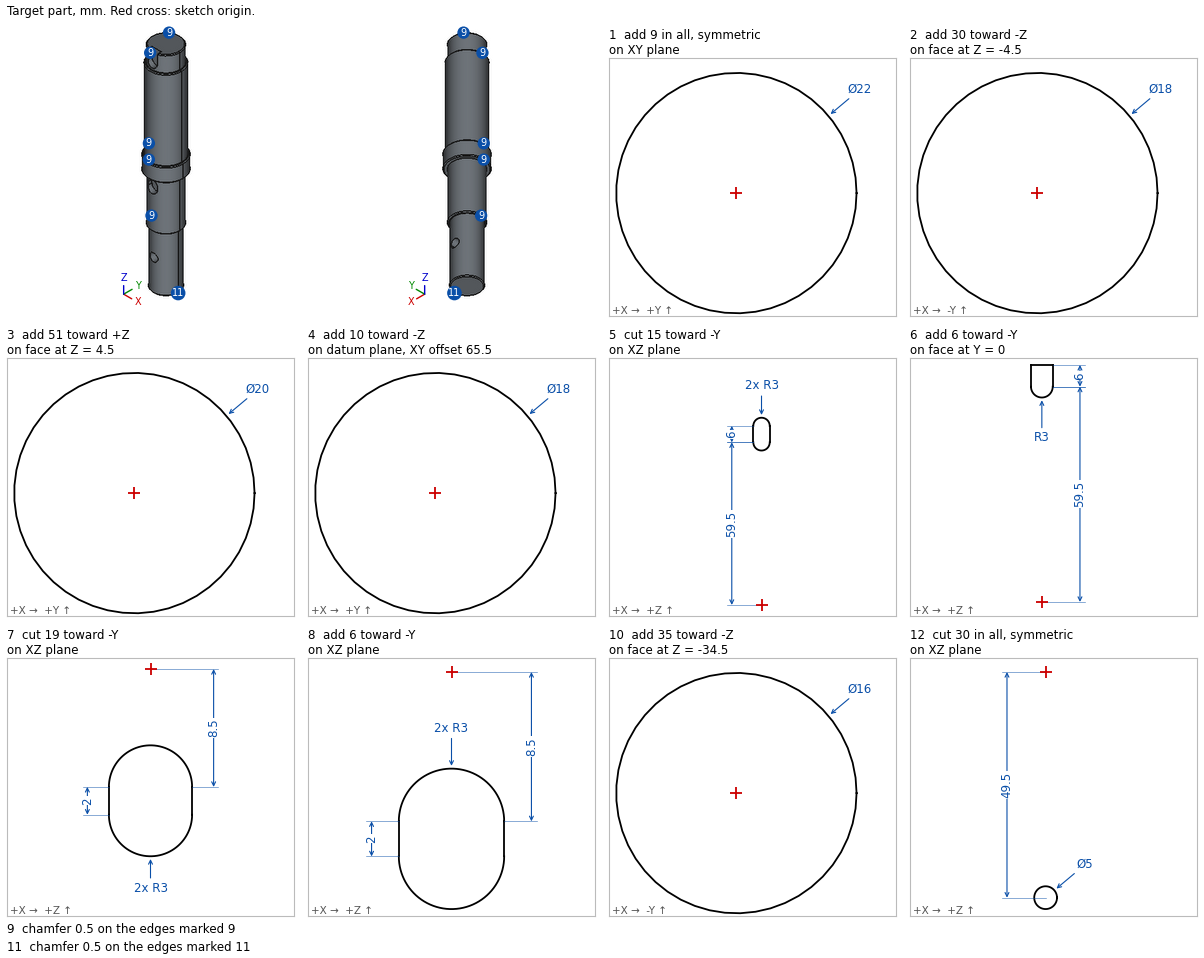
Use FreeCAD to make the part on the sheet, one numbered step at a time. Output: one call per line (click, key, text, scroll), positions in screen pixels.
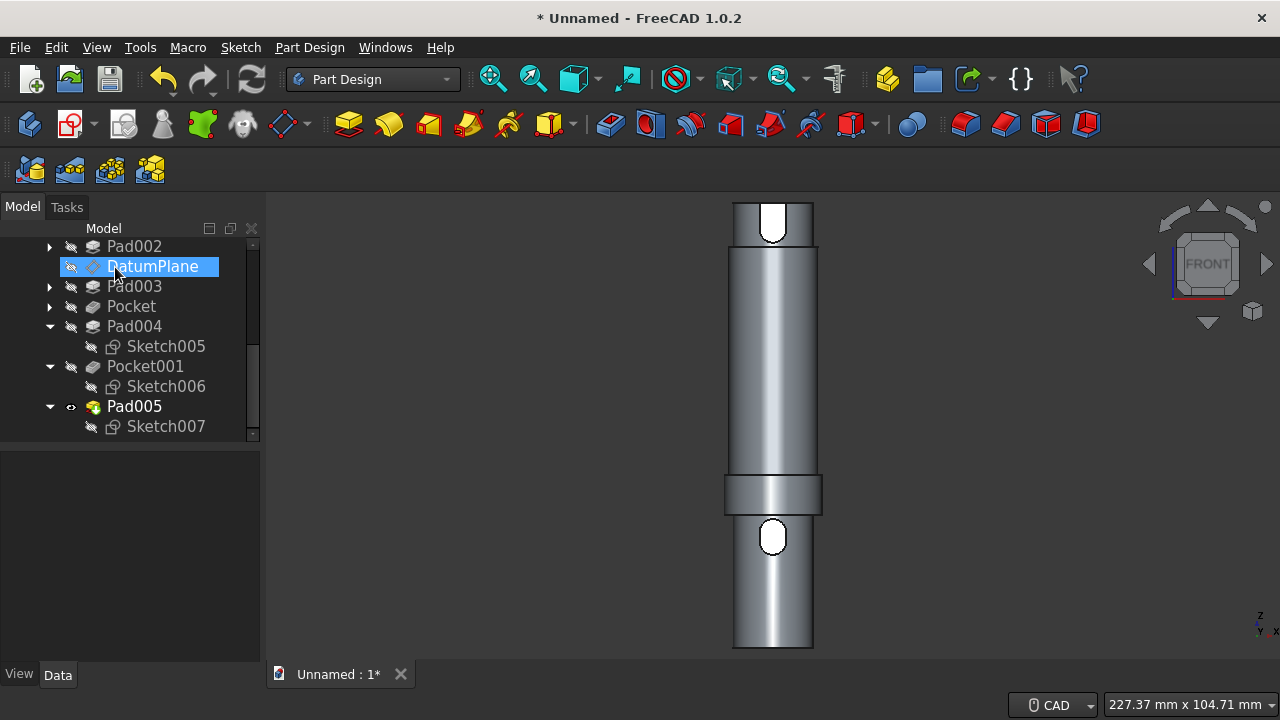
click(737, 246)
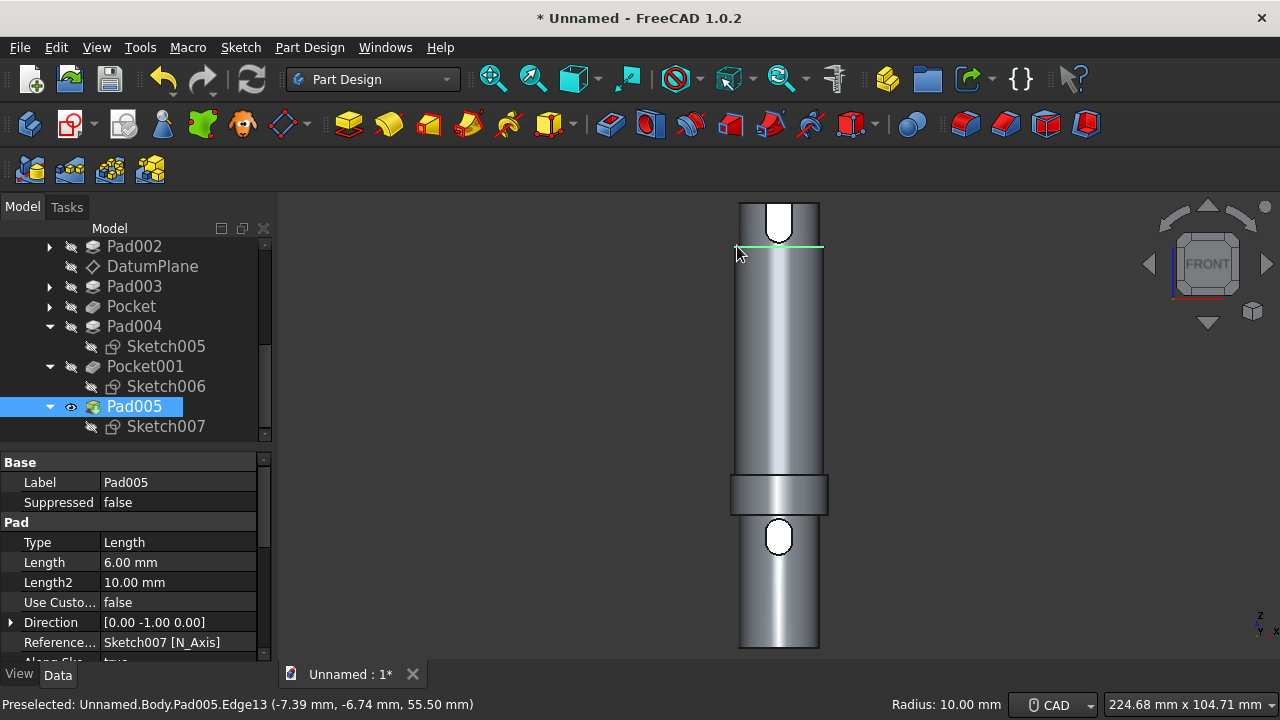
click(739, 514, ctrl)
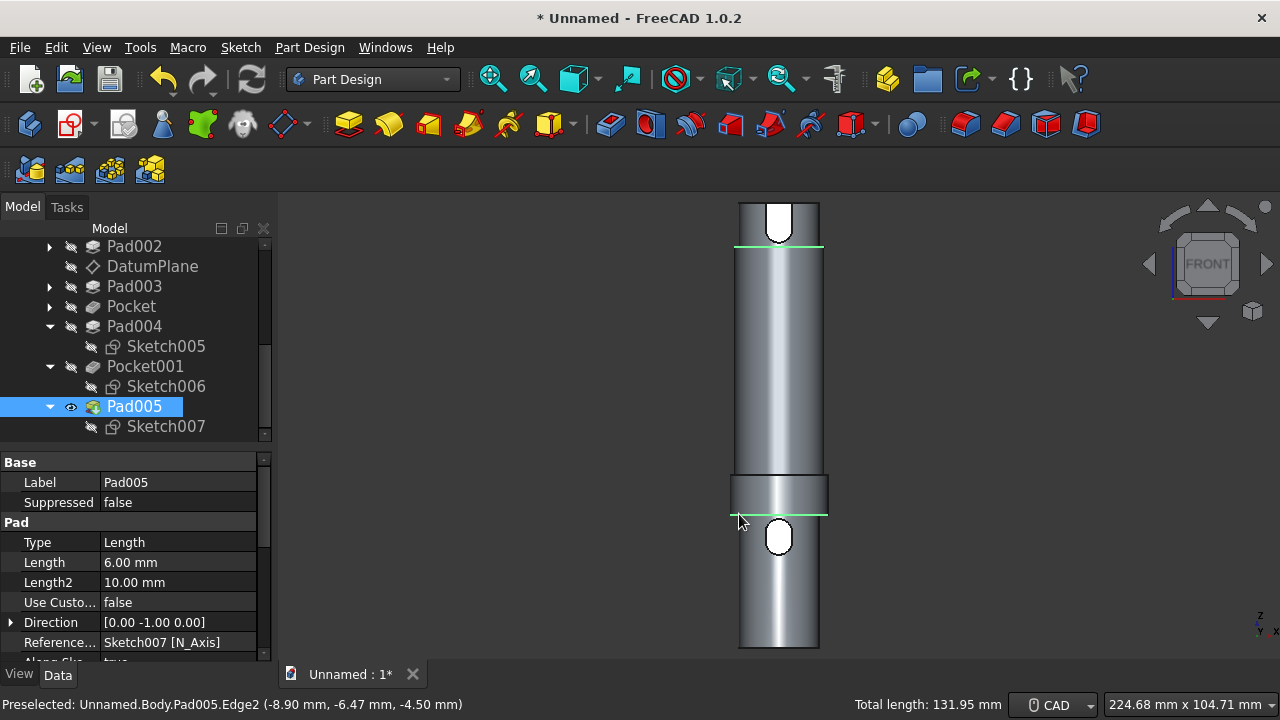
click(739, 474, ctrl)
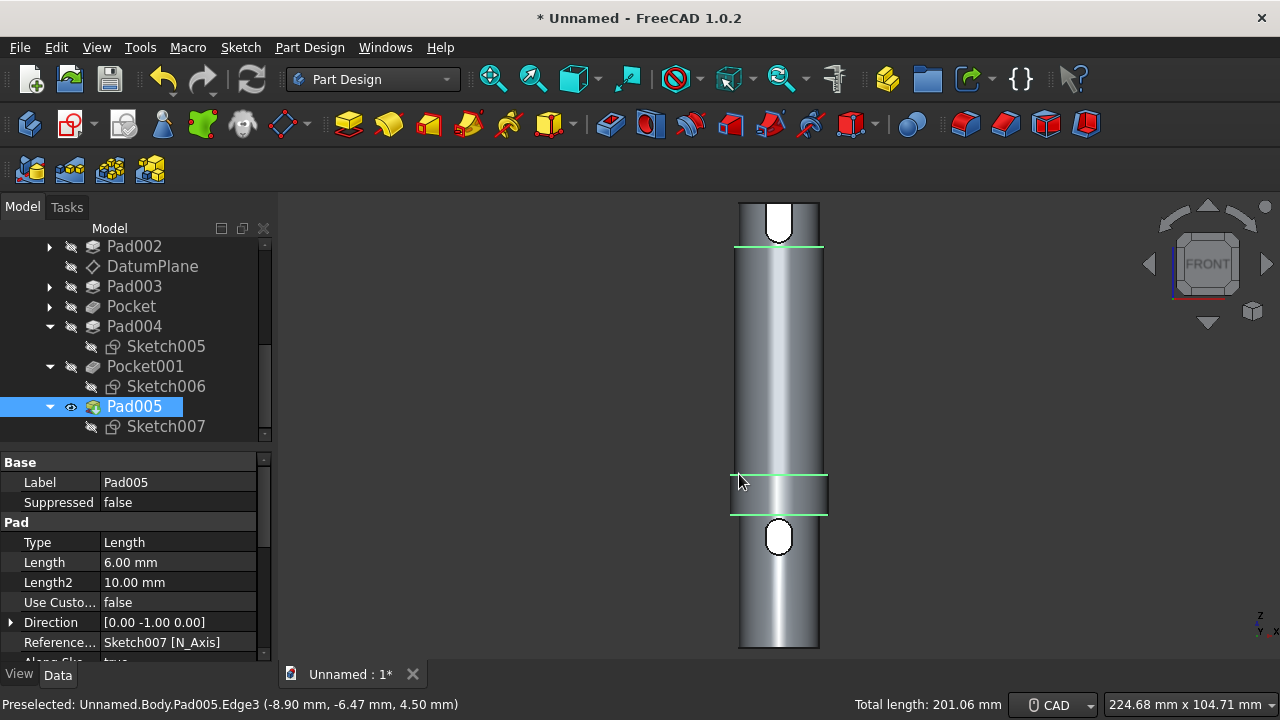
key(0)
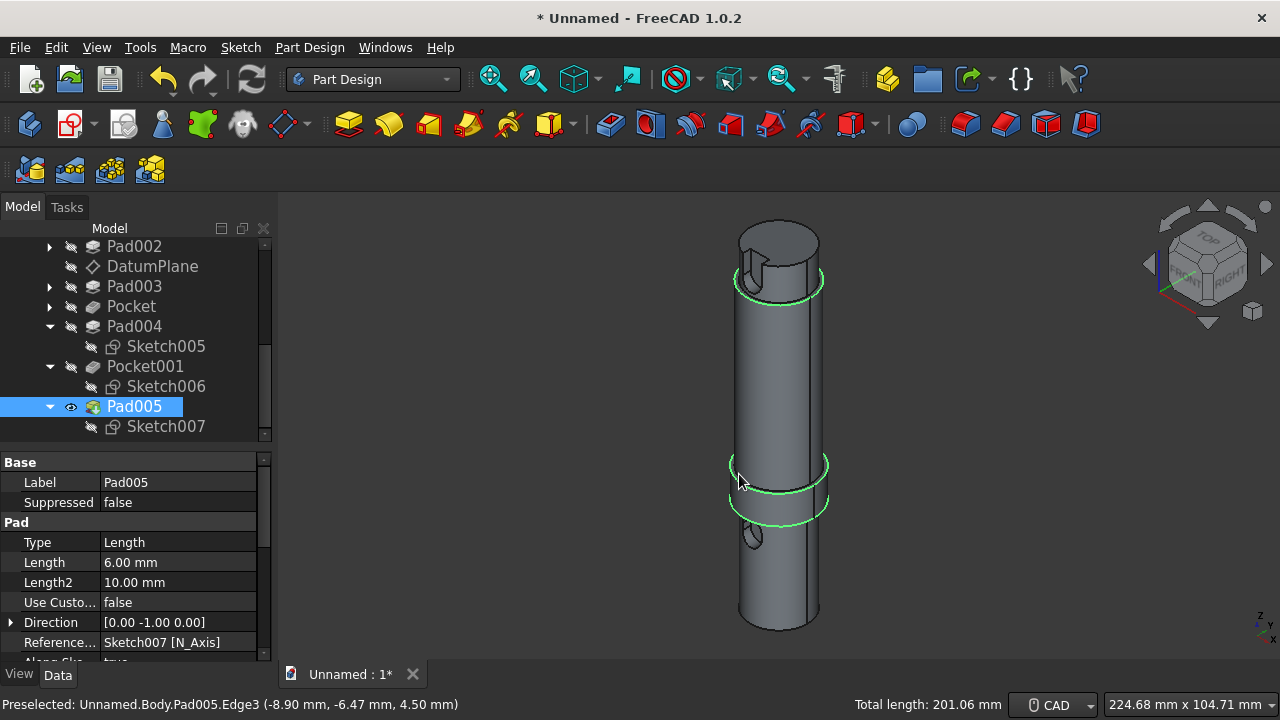
click(814, 231, ctrl)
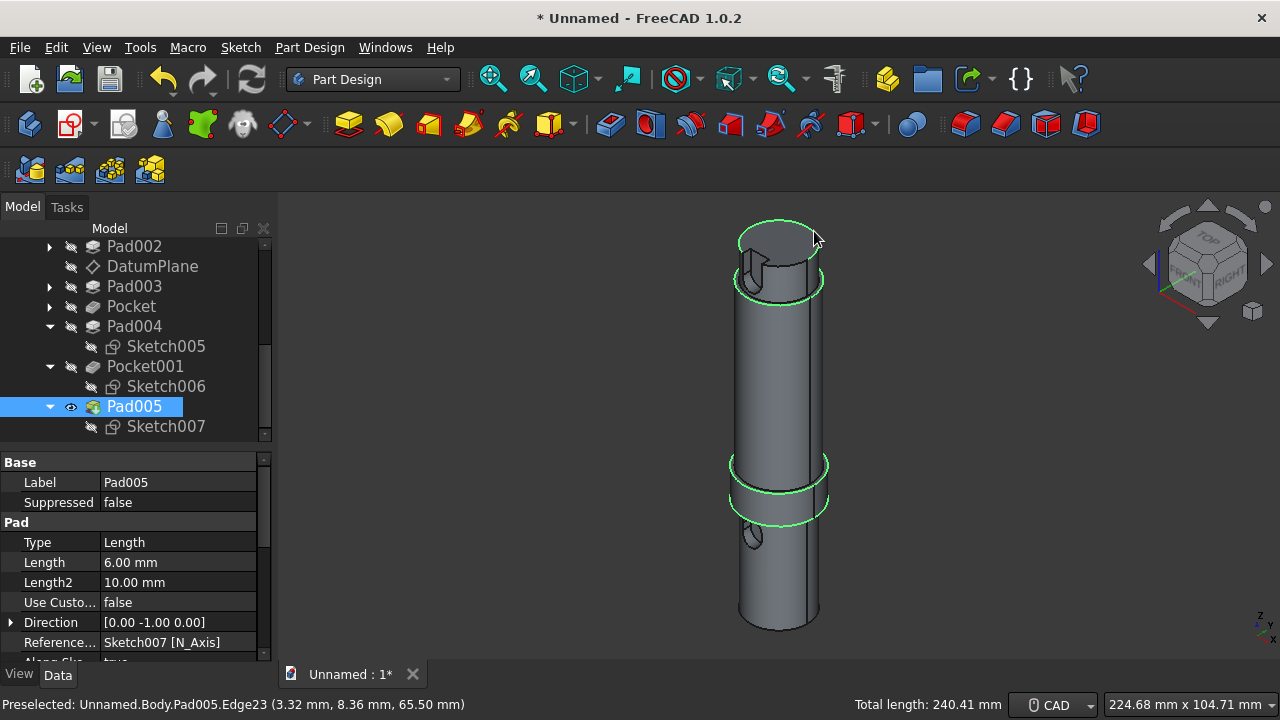
click(743, 617, ctrl)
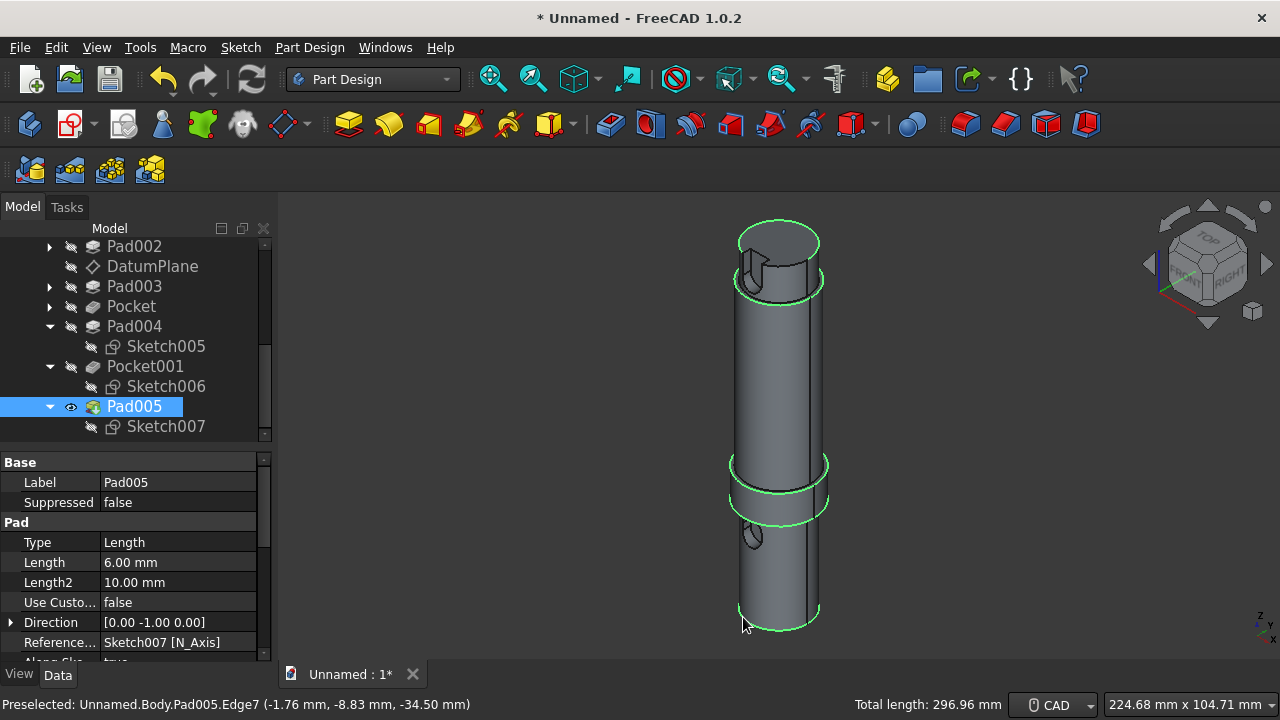
click(1006, 124)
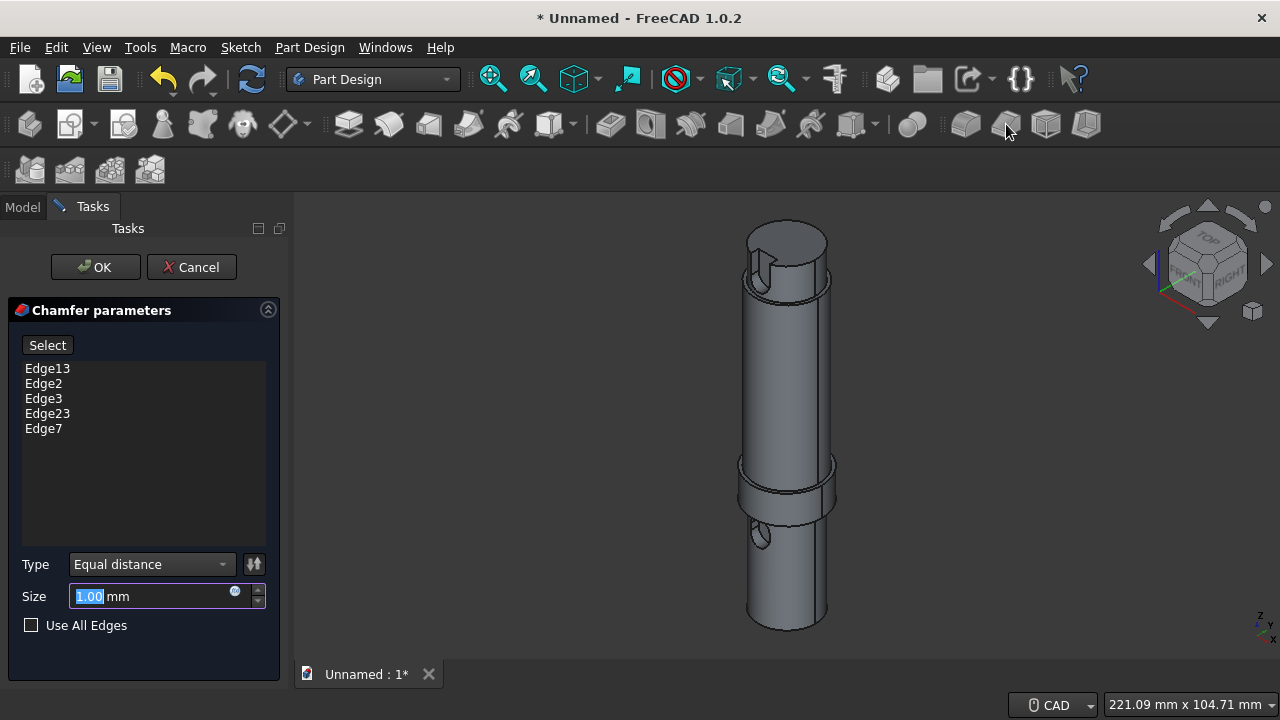
text(0.5)
key(Tab)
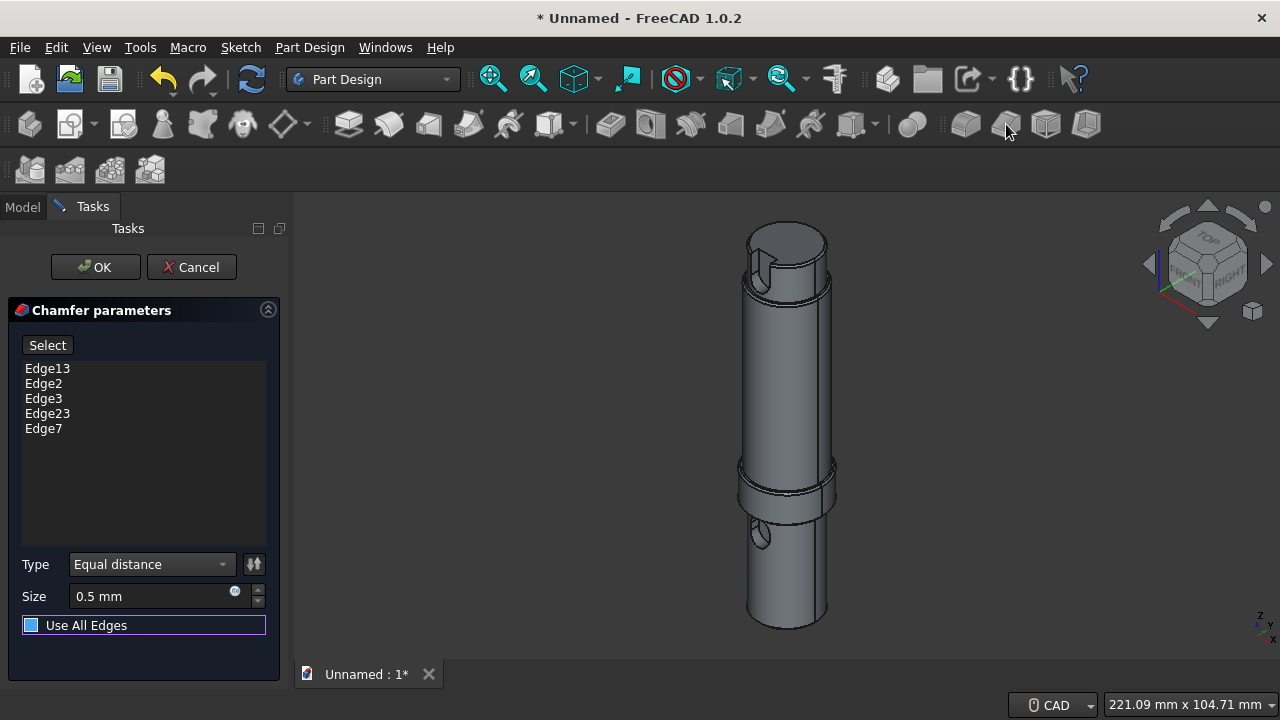
click(96, 267)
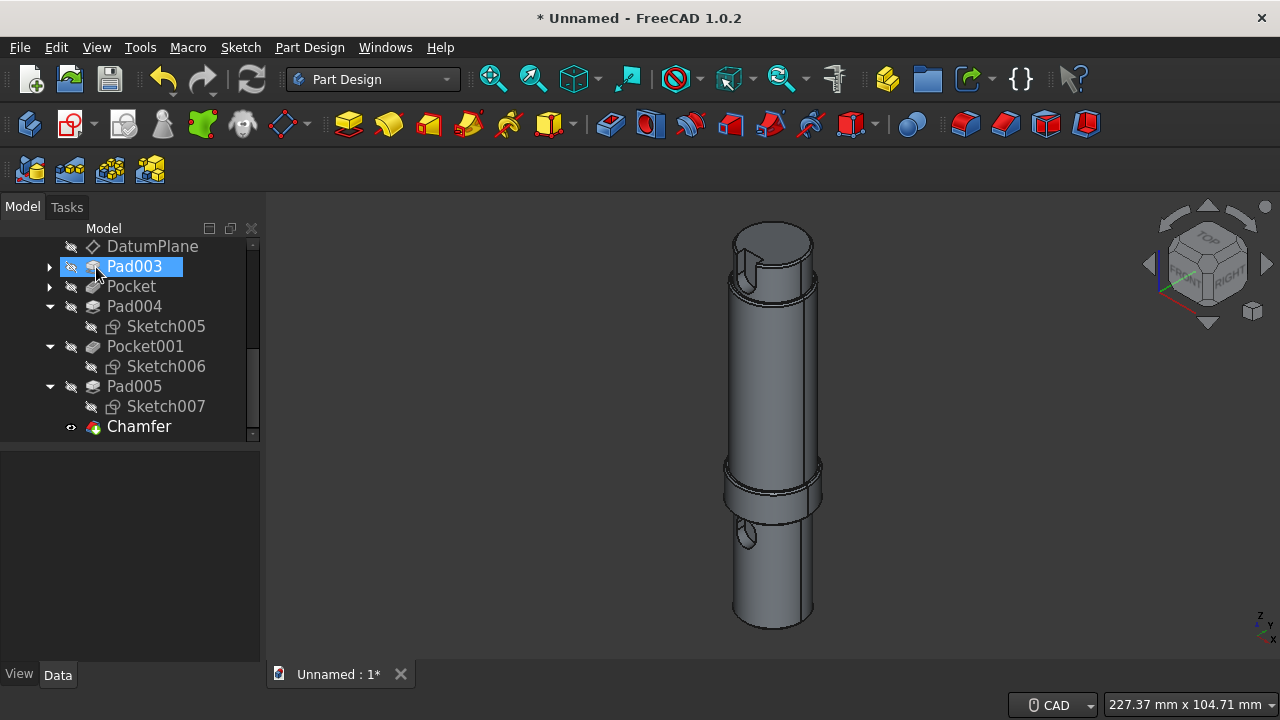
key(5)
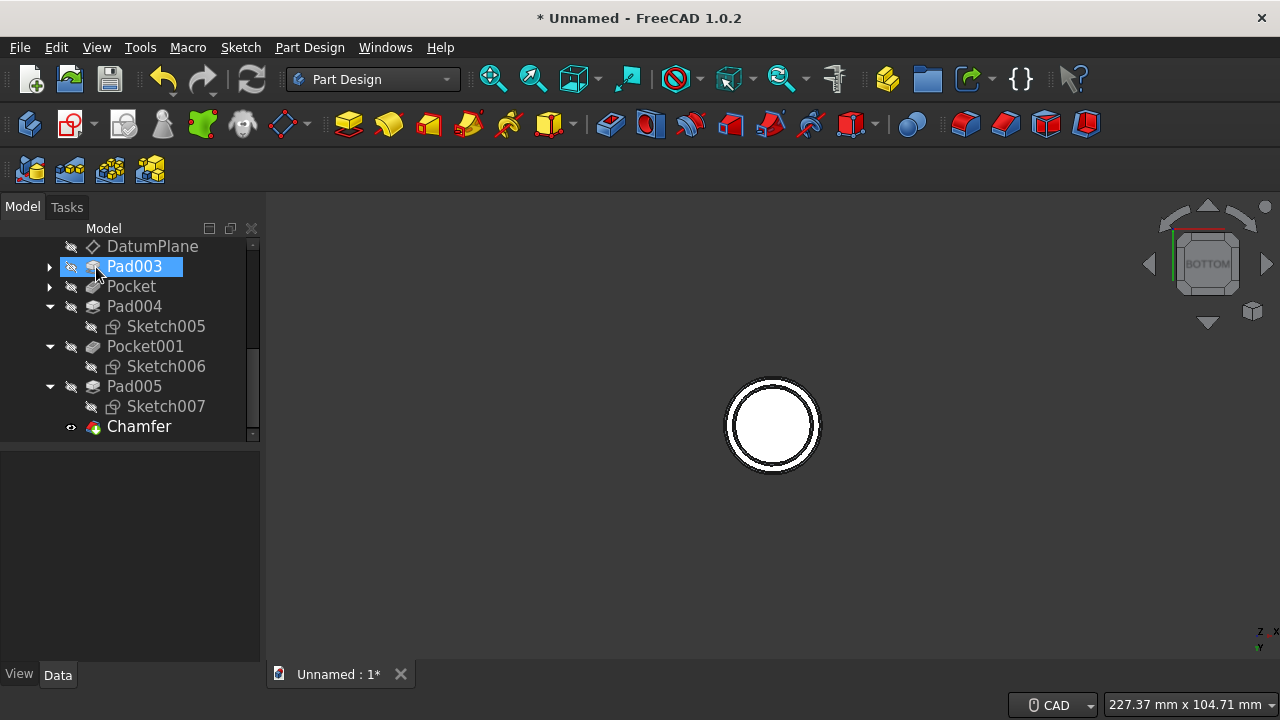
click(494, 80)